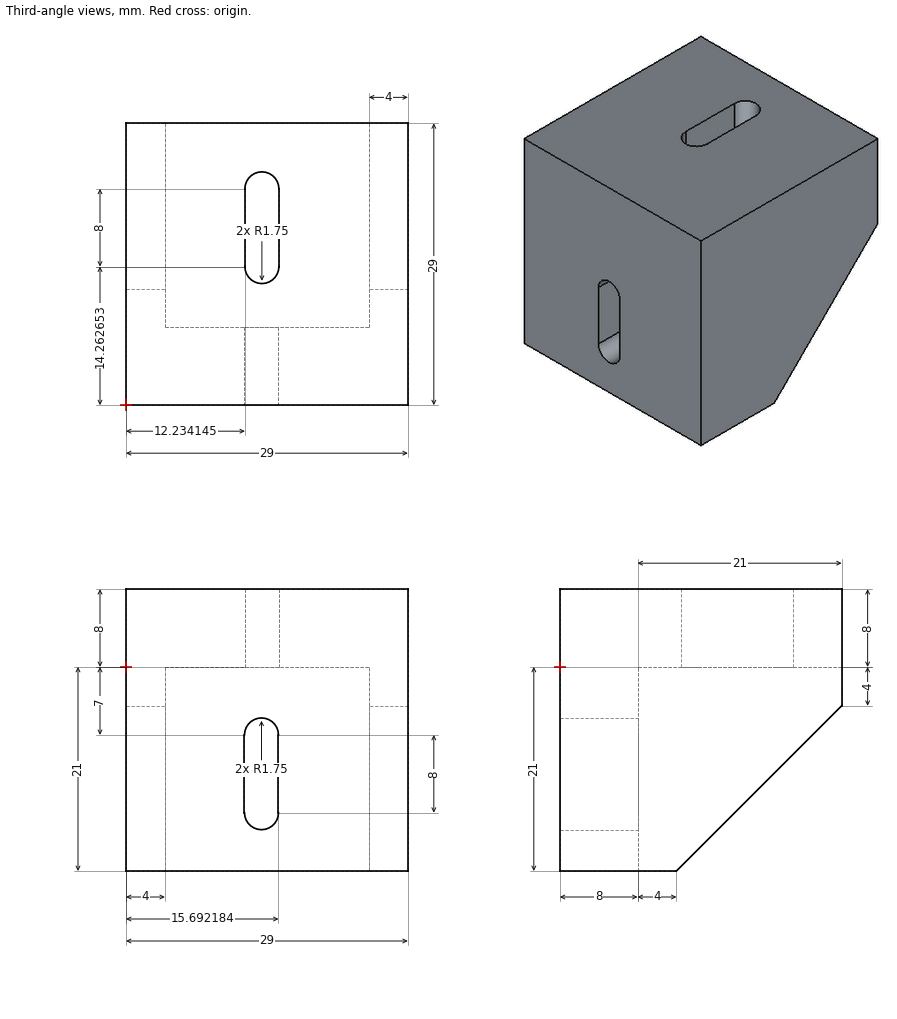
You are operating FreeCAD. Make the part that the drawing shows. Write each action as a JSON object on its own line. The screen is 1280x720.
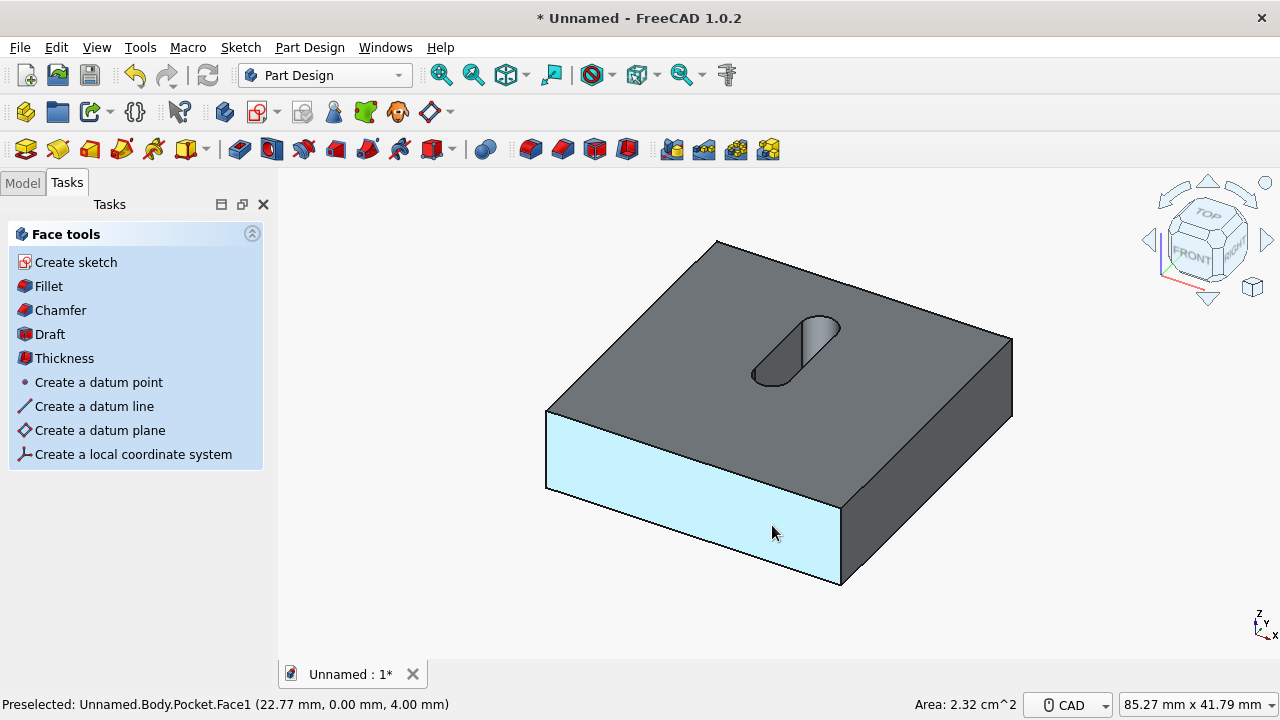
{"action": "left_click", "coordinate": [258, 112]}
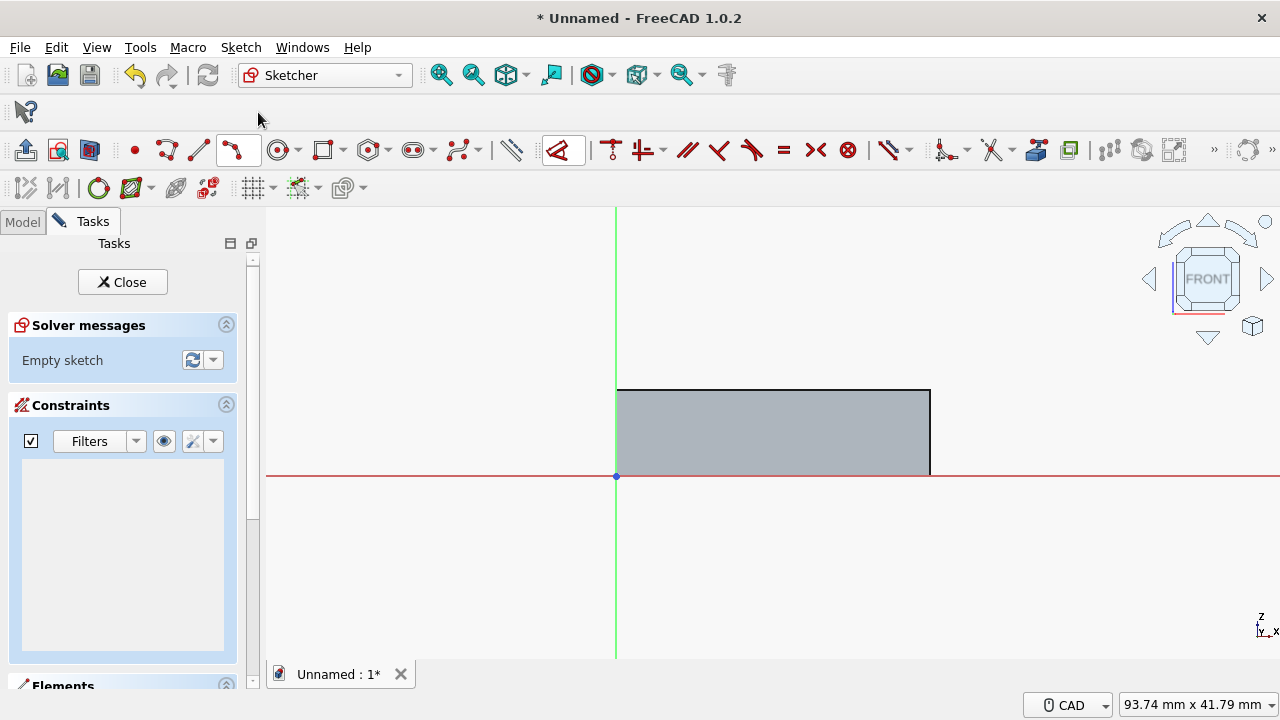
{"action": "scroll", "coordinate": [565, 235], "scroll_direction": "down", "scroll_amount": 2}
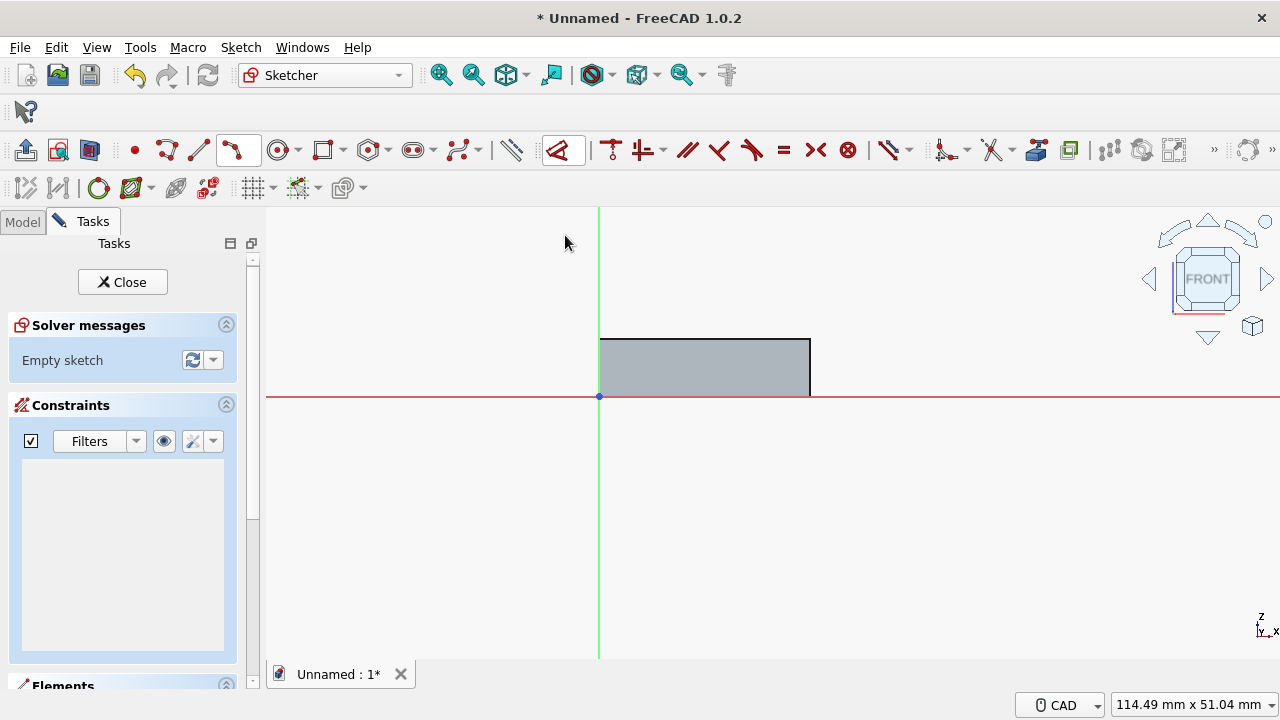
{"action": "scroll", "coordinate": [705, 521], "scroll_direction": "up", "scroll_amount": 3}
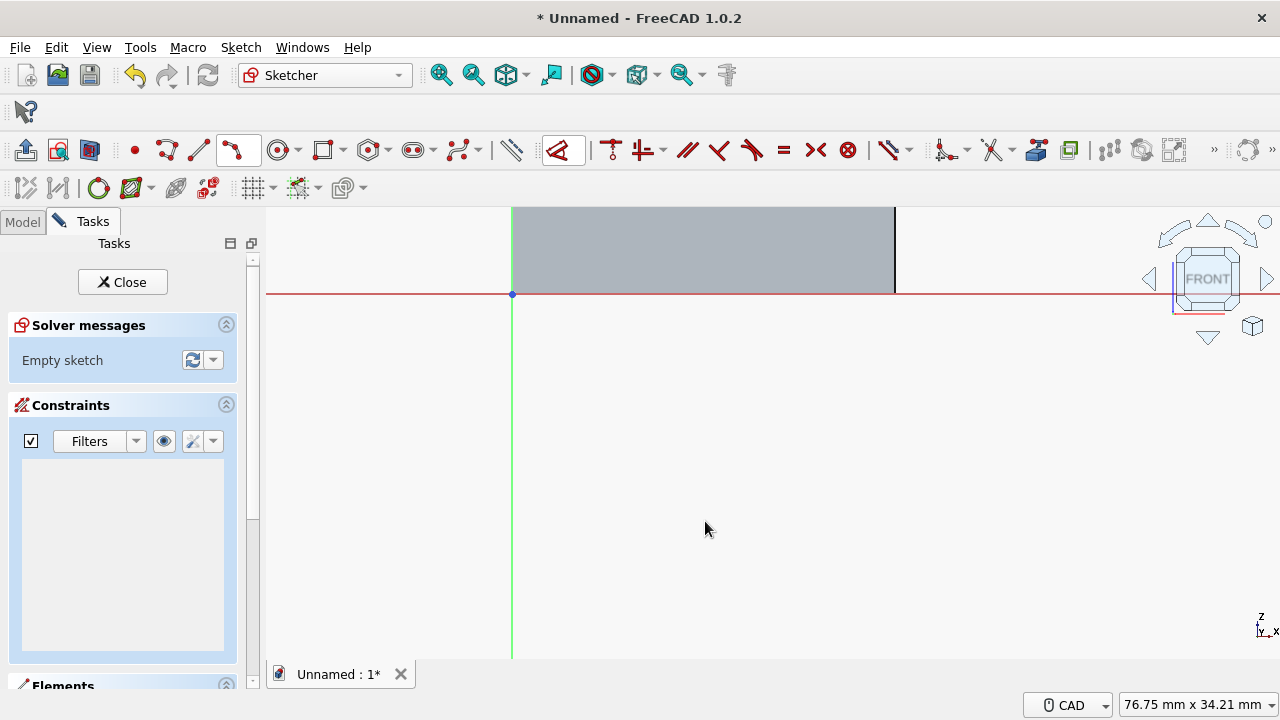
{"action": "left_click", "coordinate": [324, 150]}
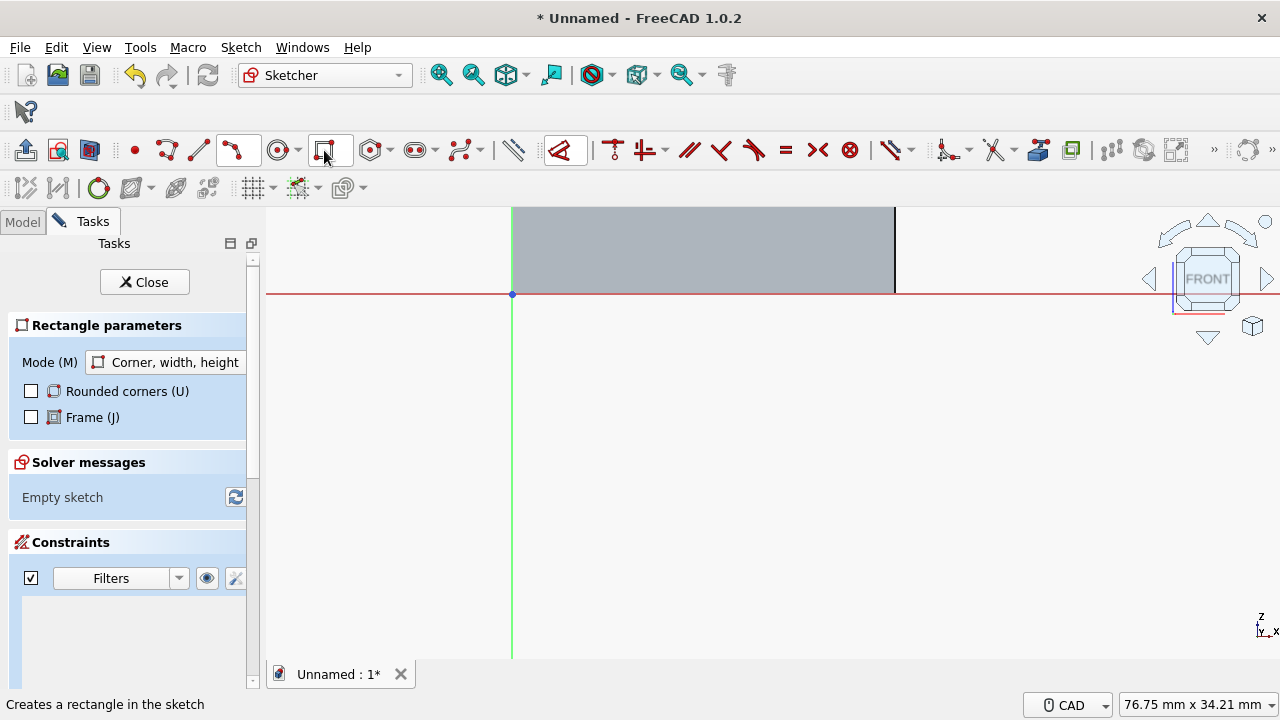
{"action": "left_click", "coordinate": [512, 294]}
{"action": "left_click", "coordinate": [895, 571]}
{"action": "key", "text": "Escape"}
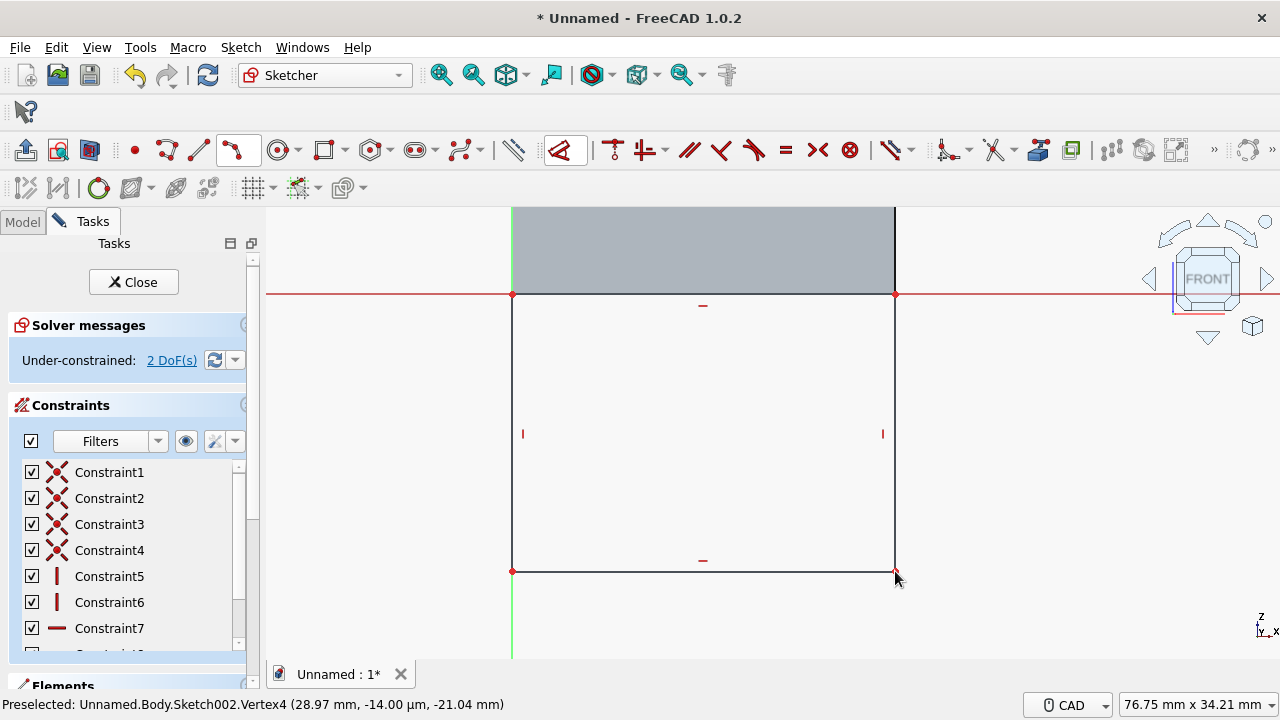
{"action": "left_click", "coordinate": [512, 377]}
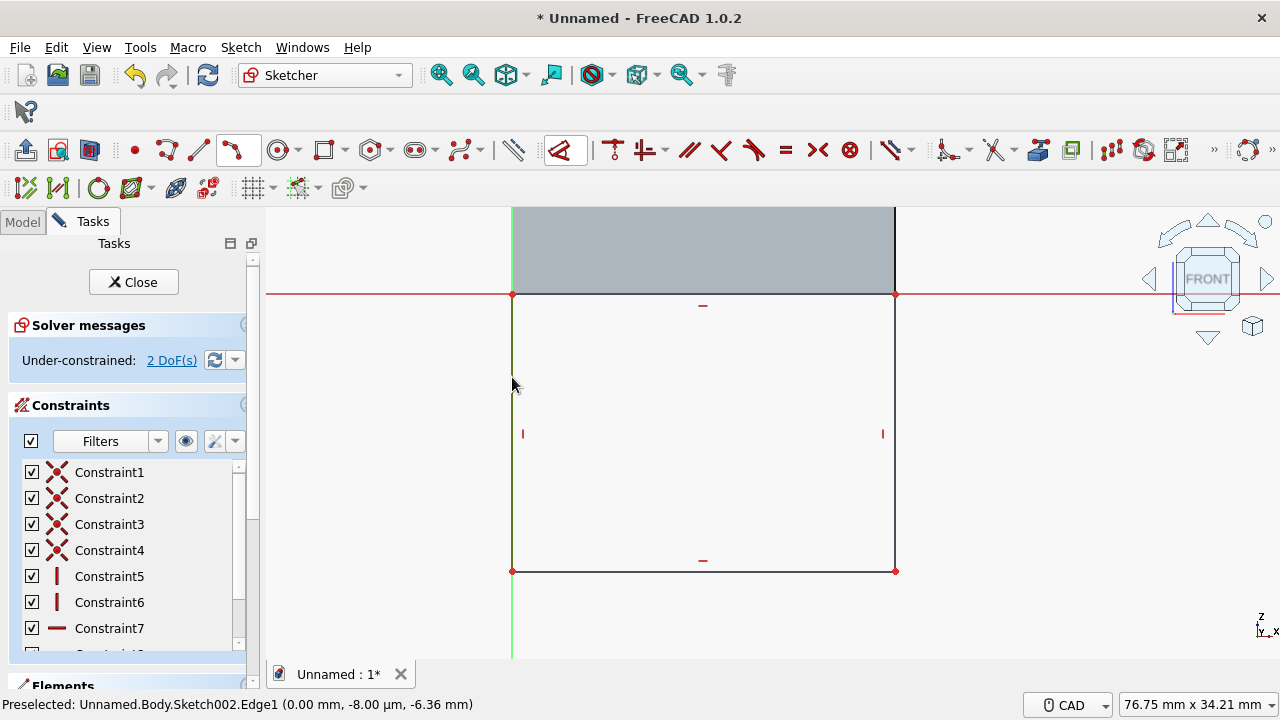
{"action": "key", "text": "i"}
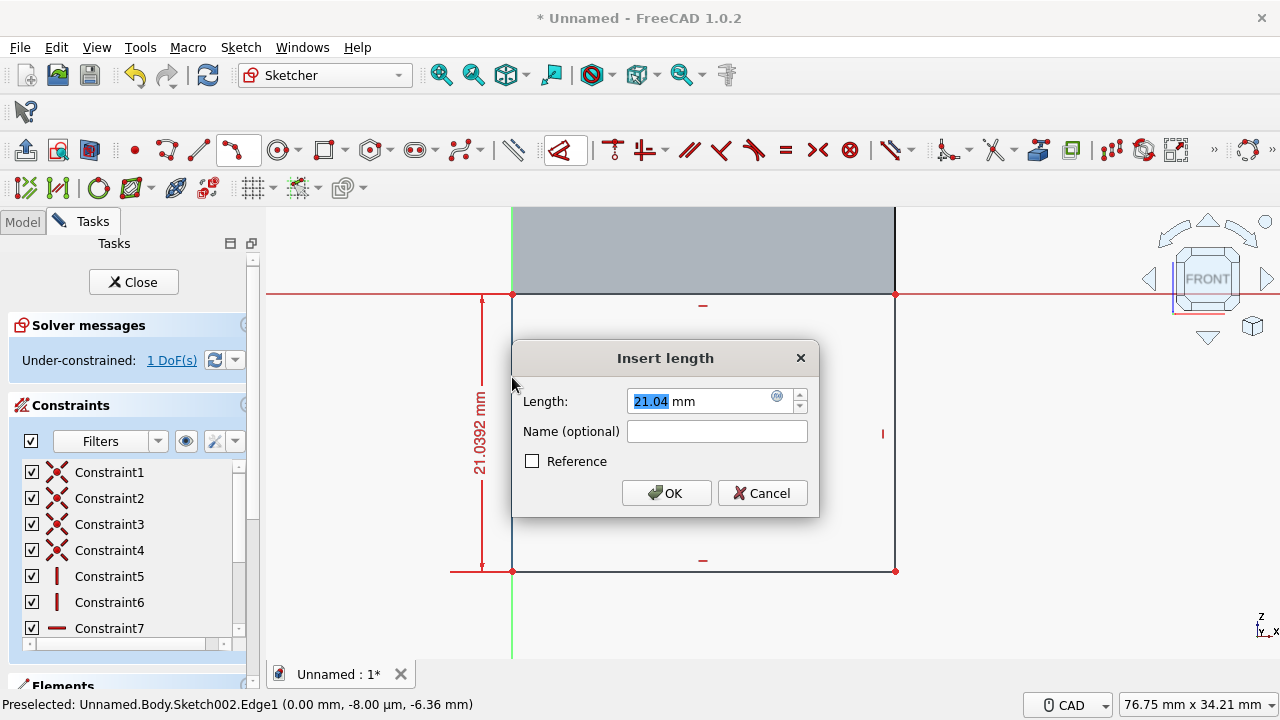
{"action": "type", "text": "21"}
{"action": "key", "text": "Return"}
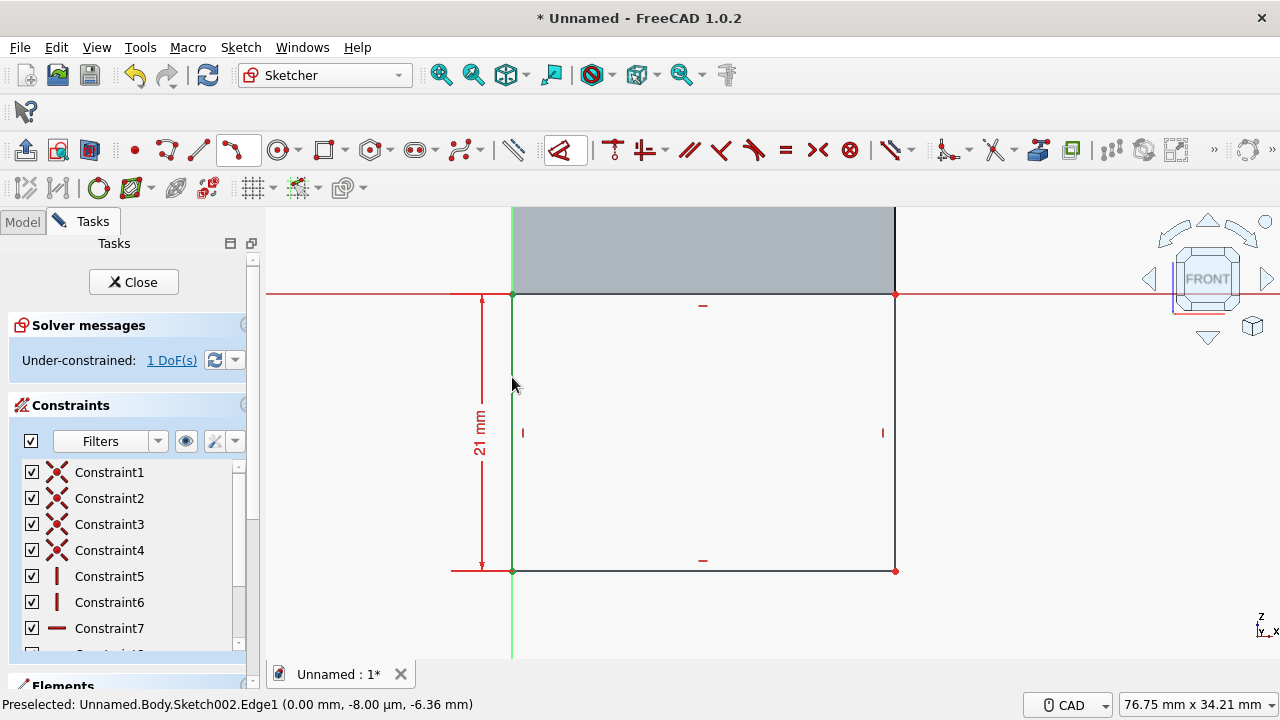
{"action": "left_click", "coordinate": [627, 571]}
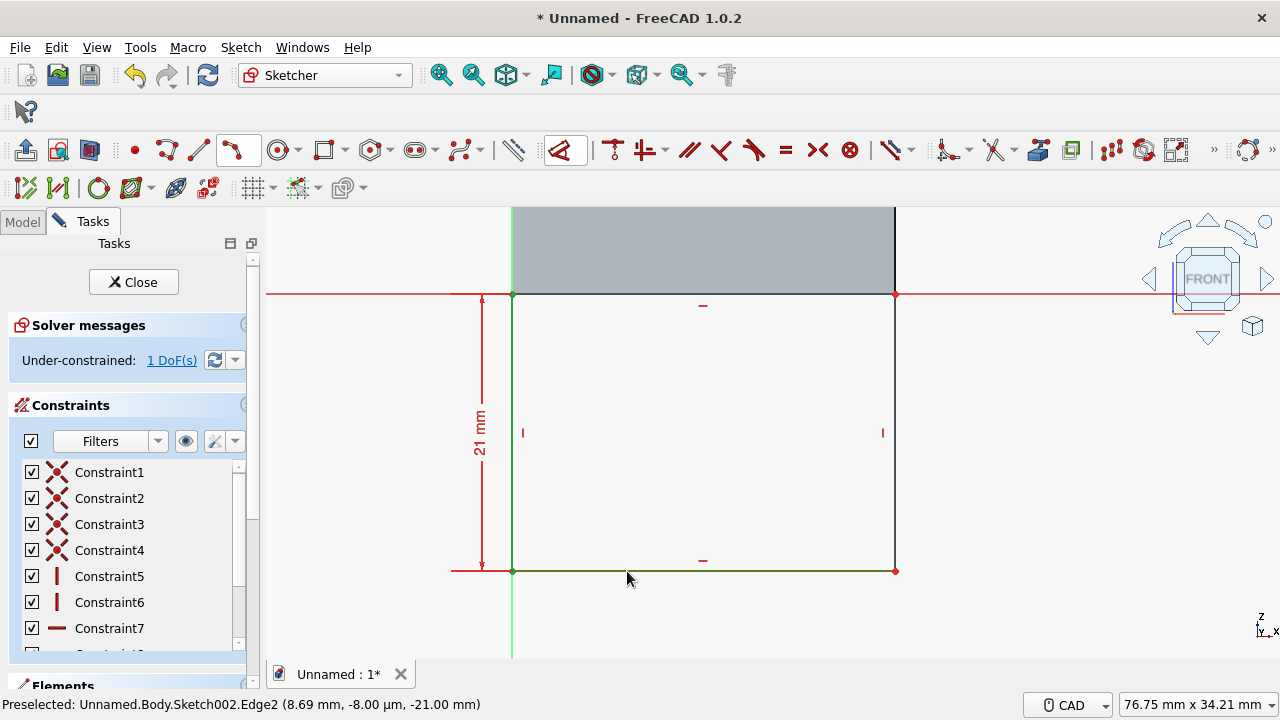
{"action": "key", "text": "l"}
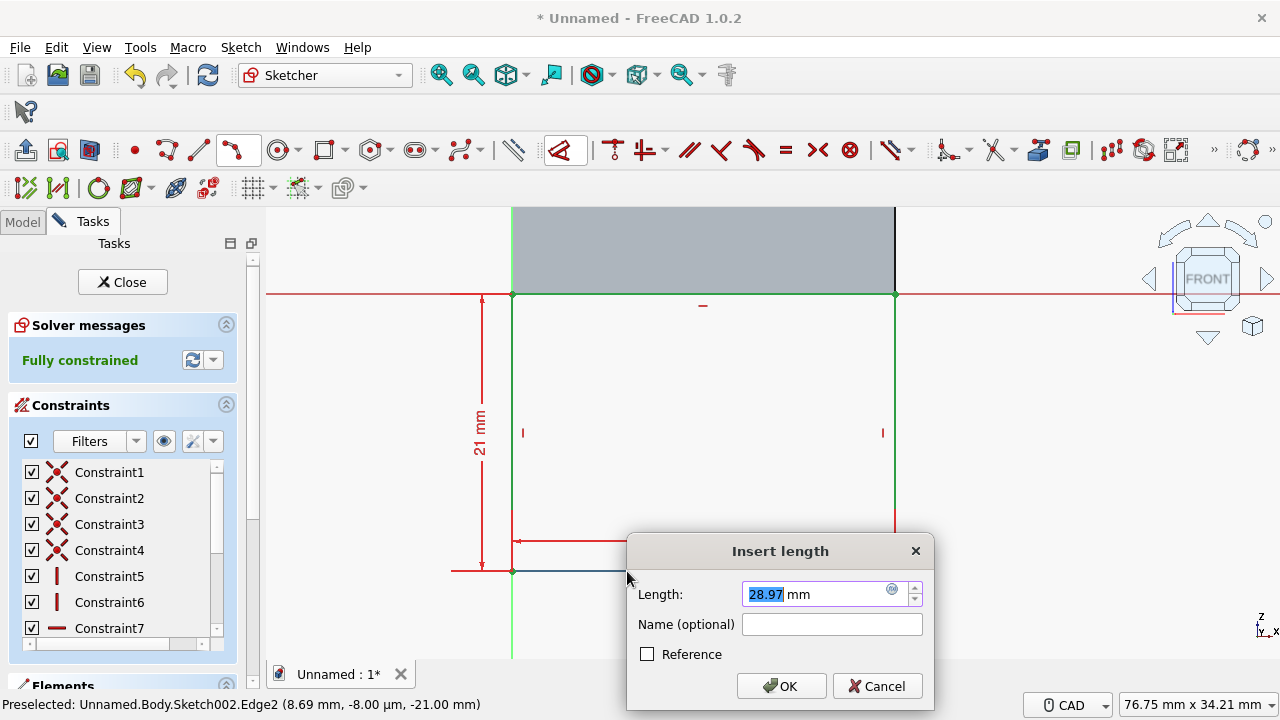
{"action": "type", "text": "29"}
{"action": "key", "text": "Return"}